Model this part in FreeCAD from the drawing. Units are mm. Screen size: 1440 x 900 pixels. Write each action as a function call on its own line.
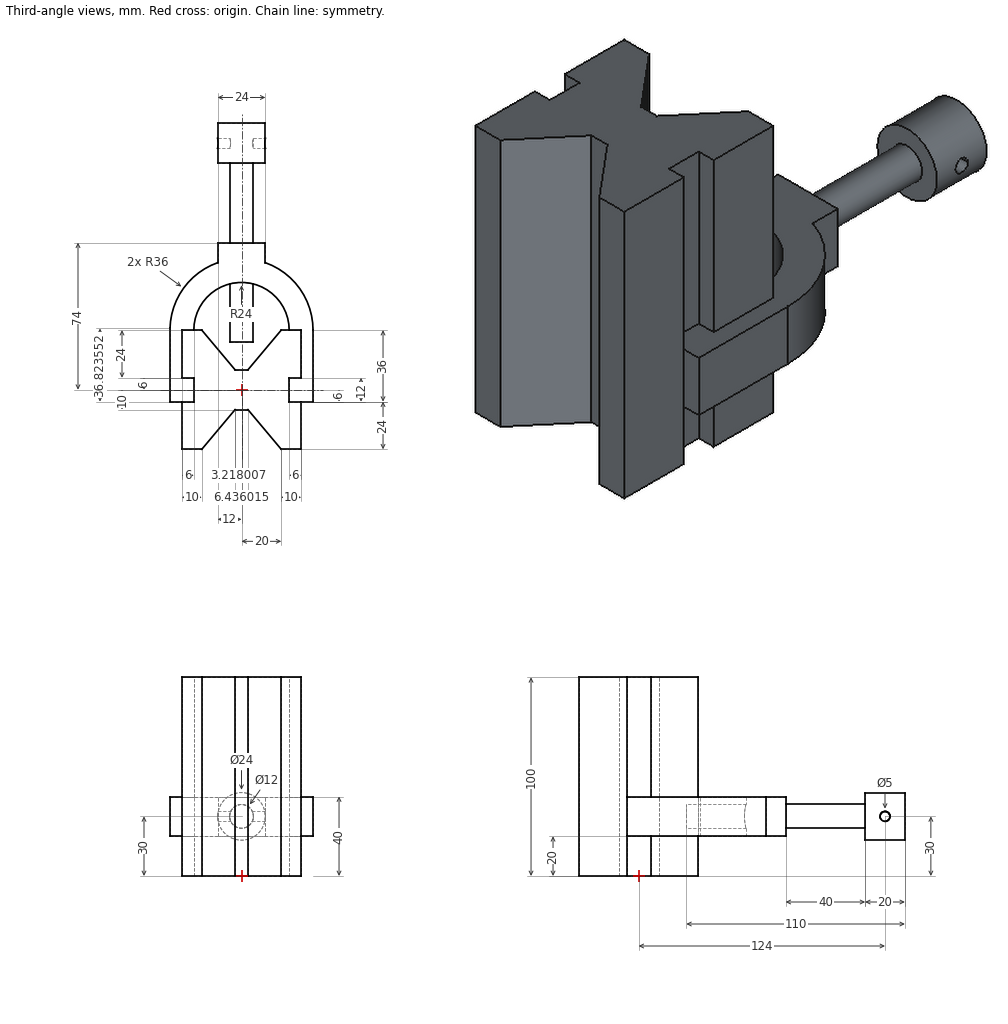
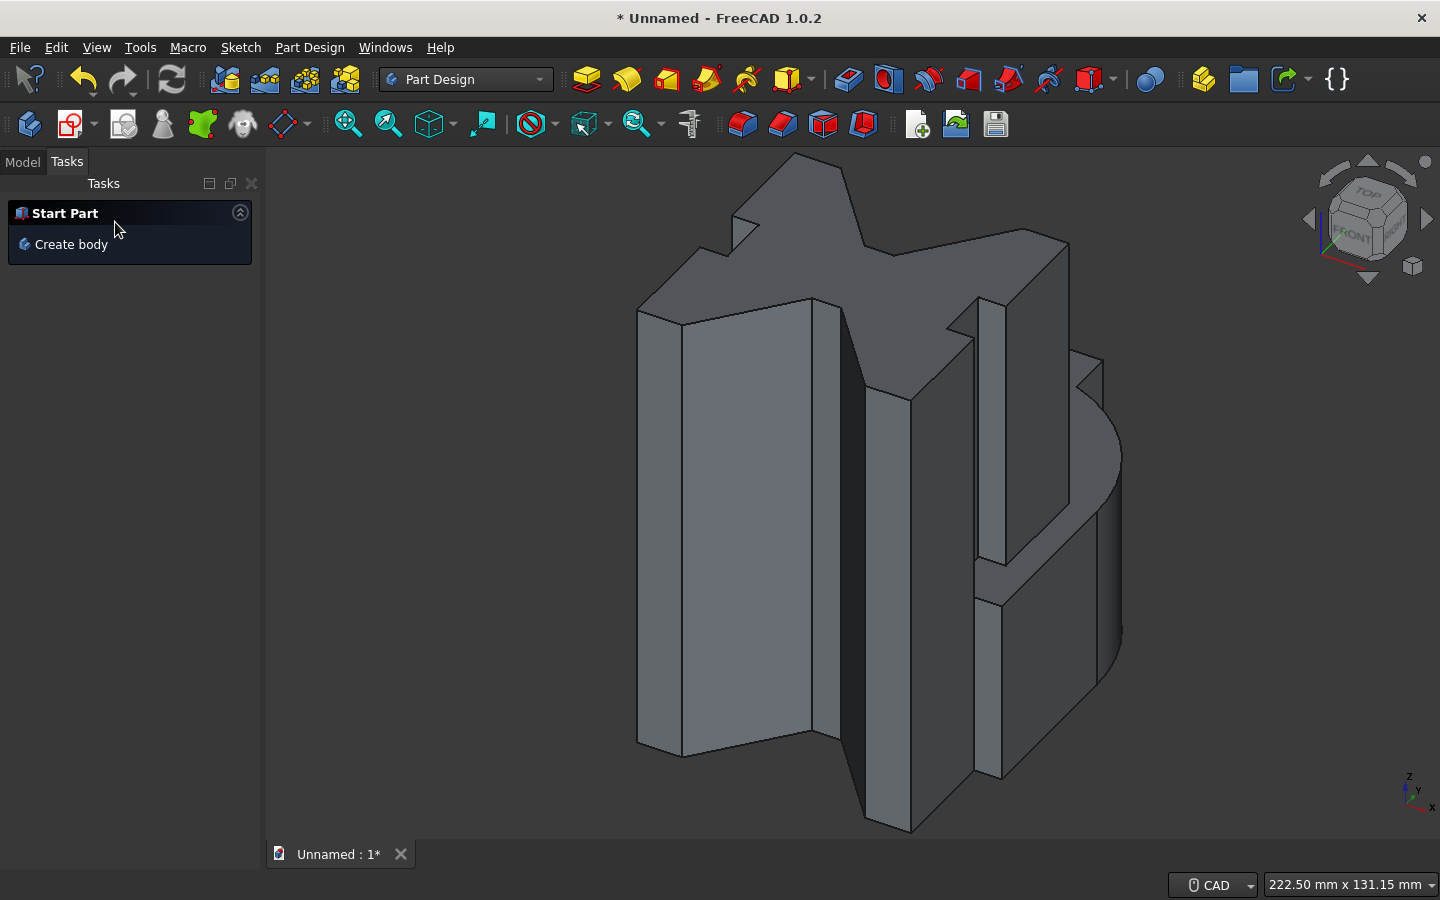
key(v)
key(f)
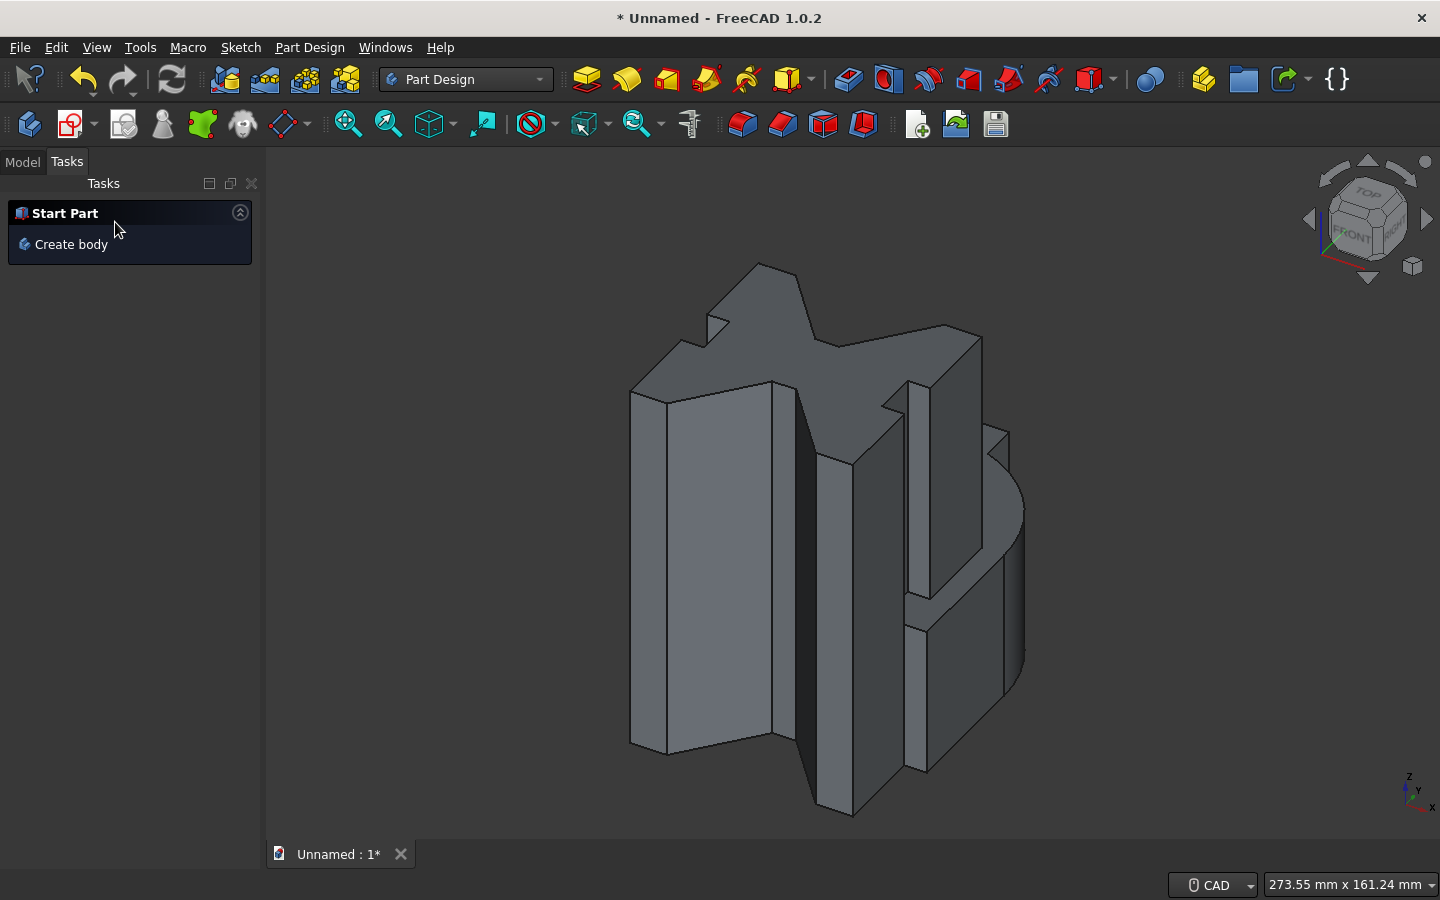
key(5)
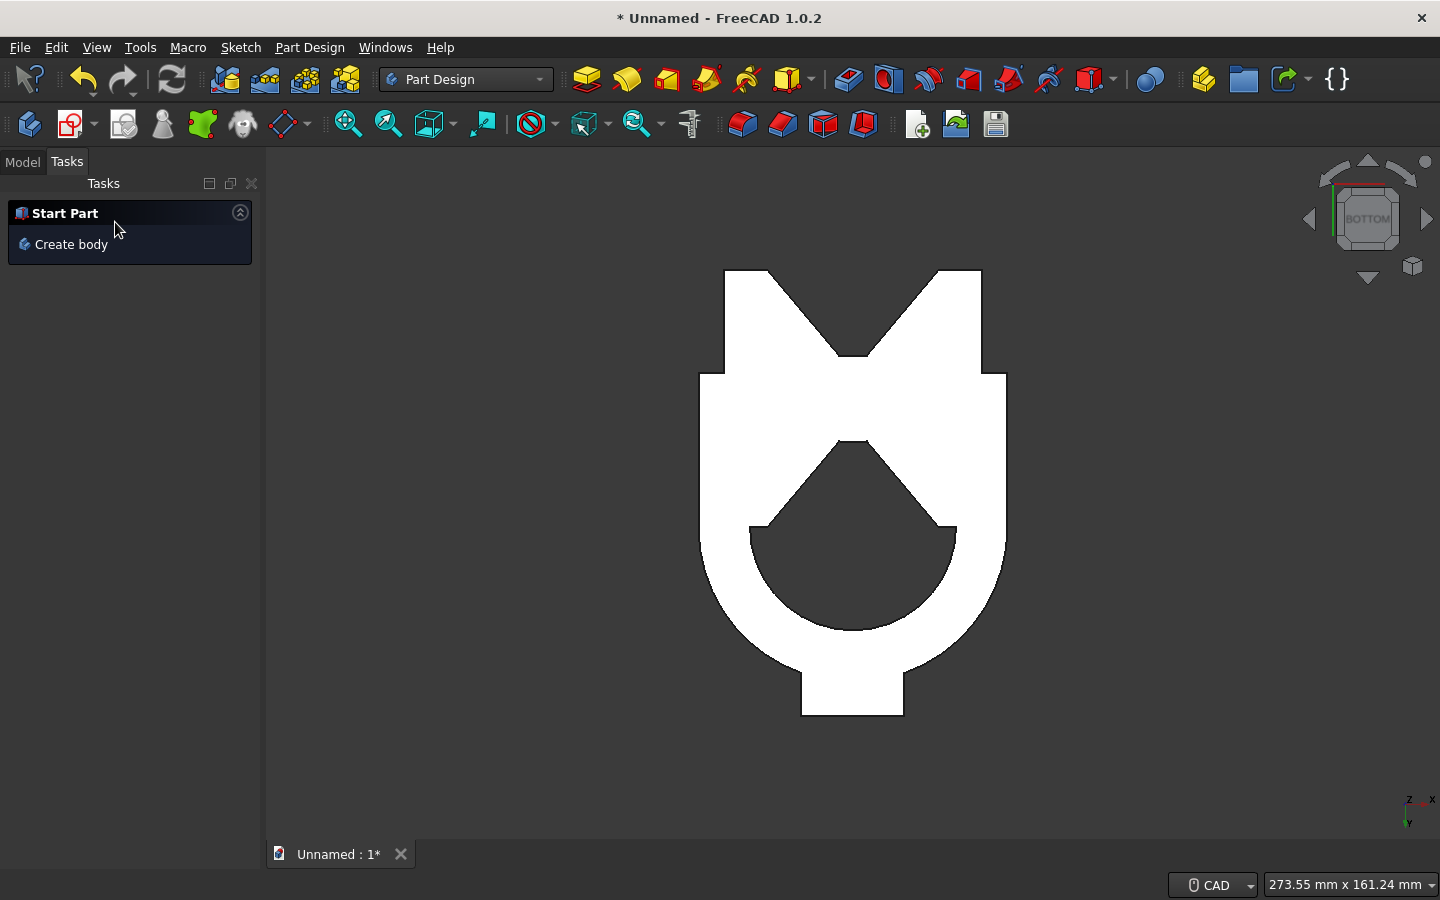
click(941, 428)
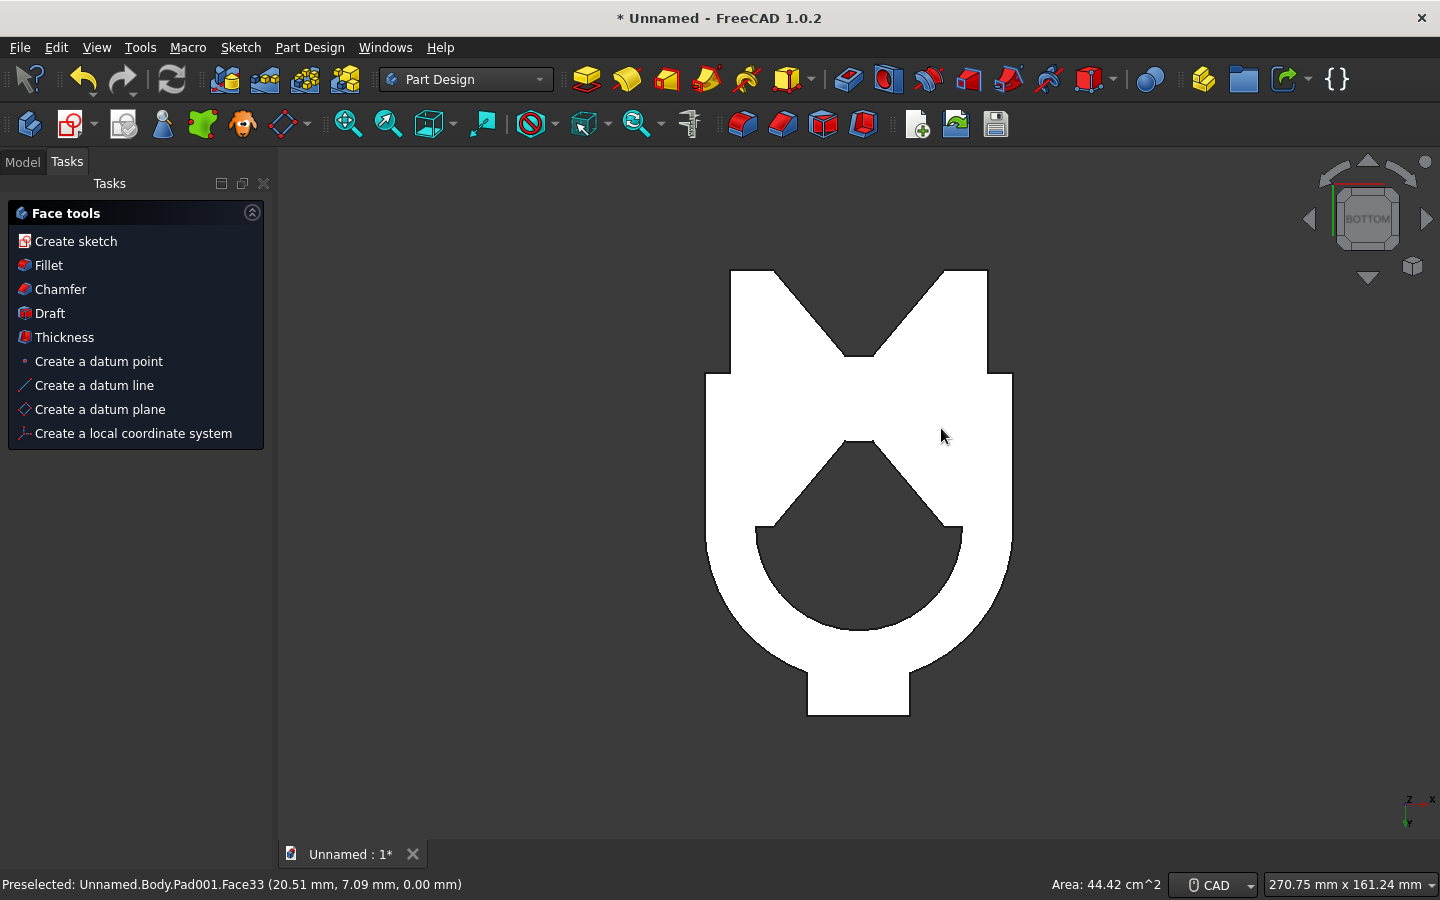
click(70, 124)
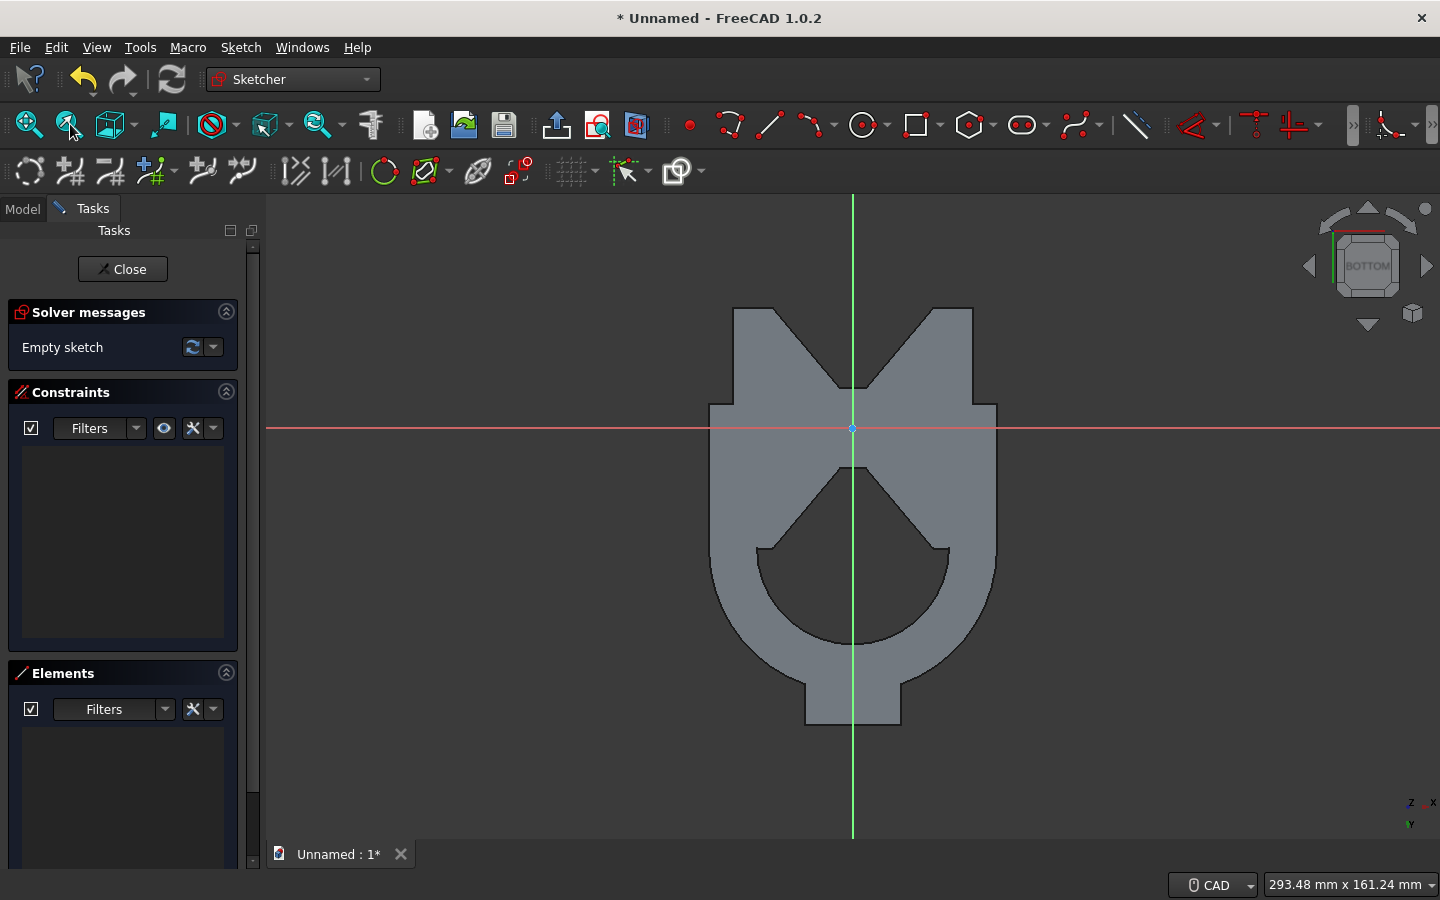
key(g)
key(m)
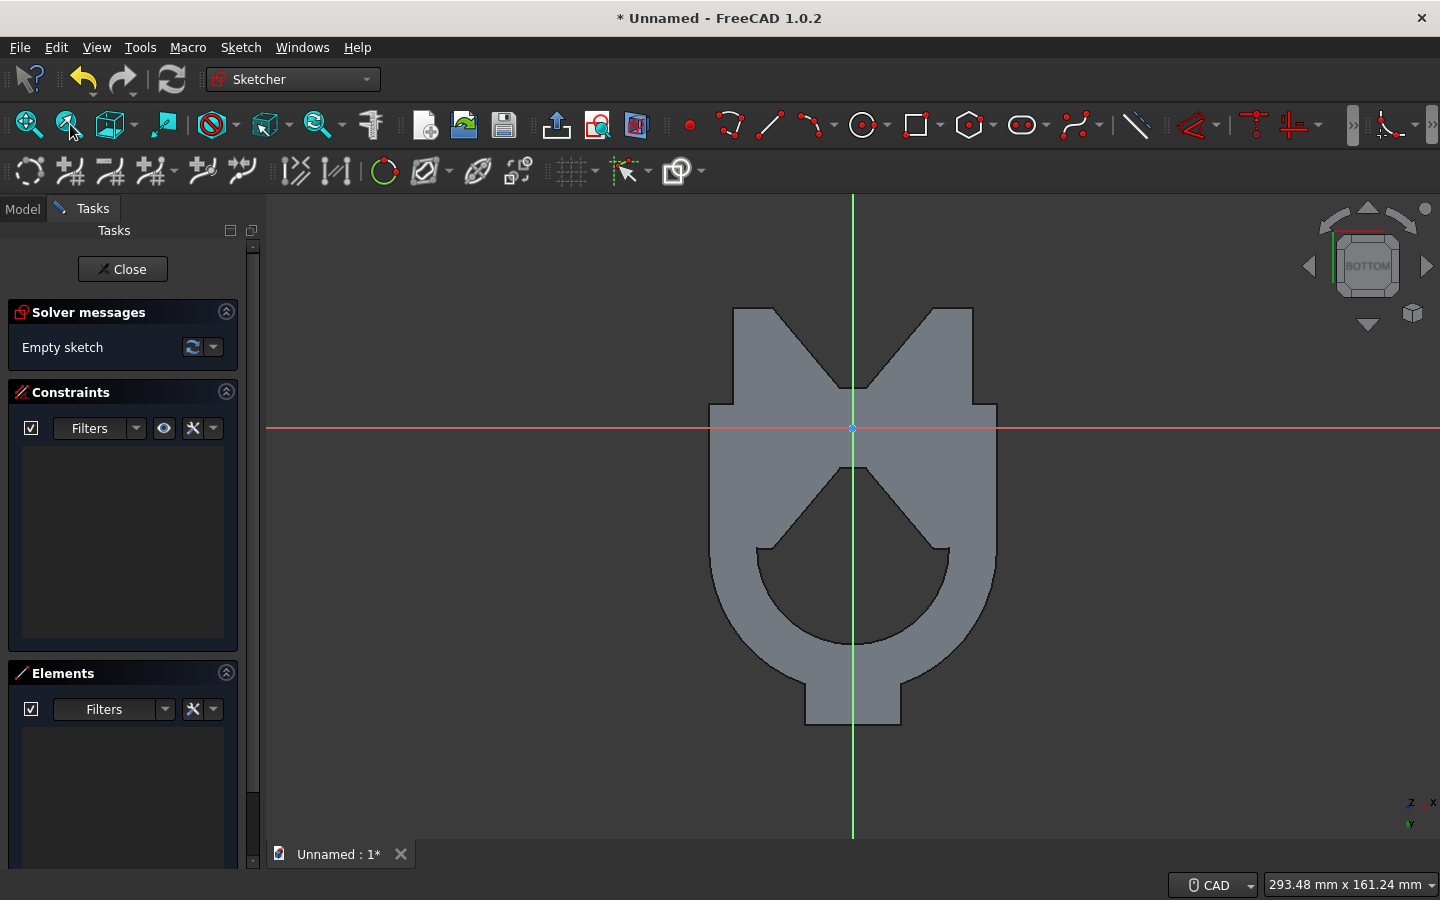
click(997, 549)
click(997, 404)
click(949, 404)
click(949, 452)
click(973, 452)
click(973, 549)
click(949, 549)
right_click(949, 549)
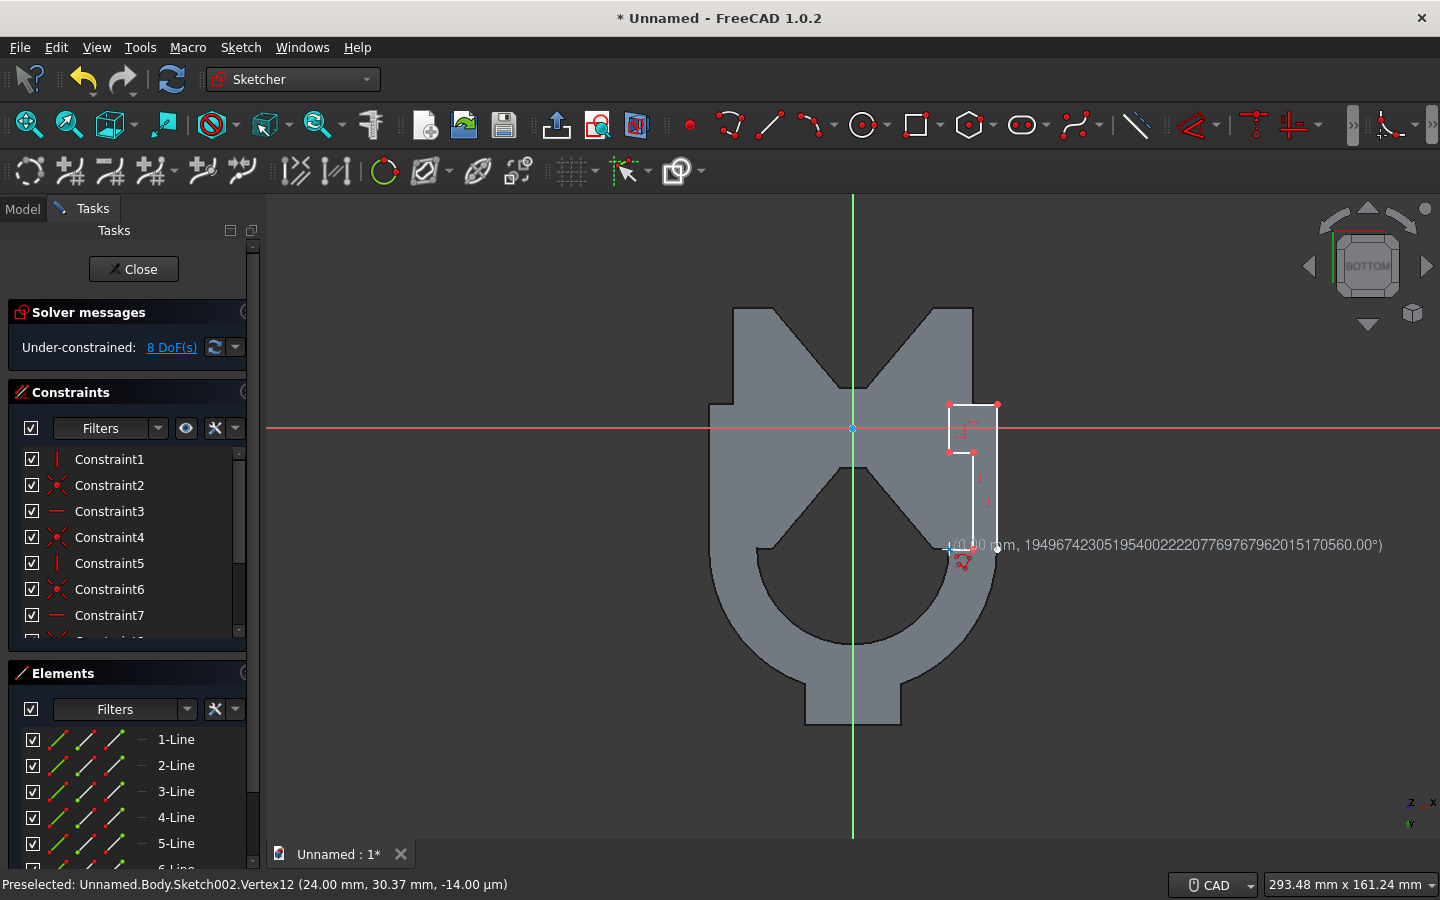
click(757, 549)
click(733, 549)
click(733, 452)
click(757, 452)
click(757, 404)
click(709, 404)
click(709, 552)
right_click(709, 552)